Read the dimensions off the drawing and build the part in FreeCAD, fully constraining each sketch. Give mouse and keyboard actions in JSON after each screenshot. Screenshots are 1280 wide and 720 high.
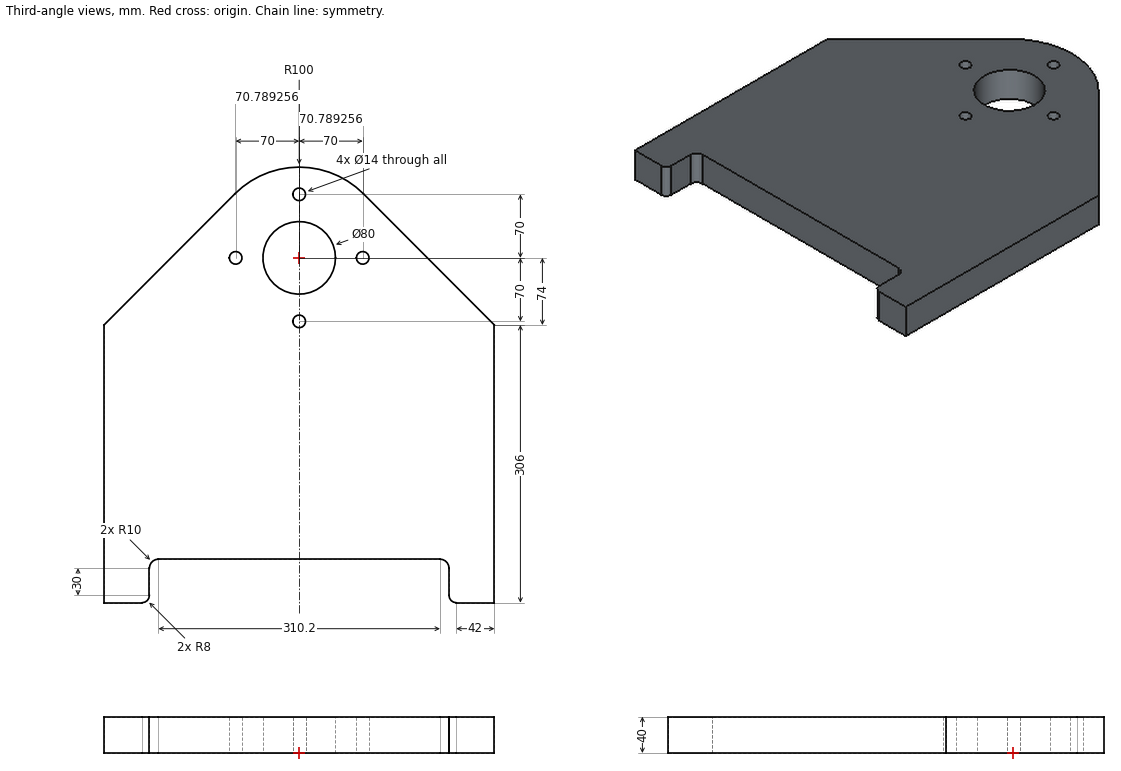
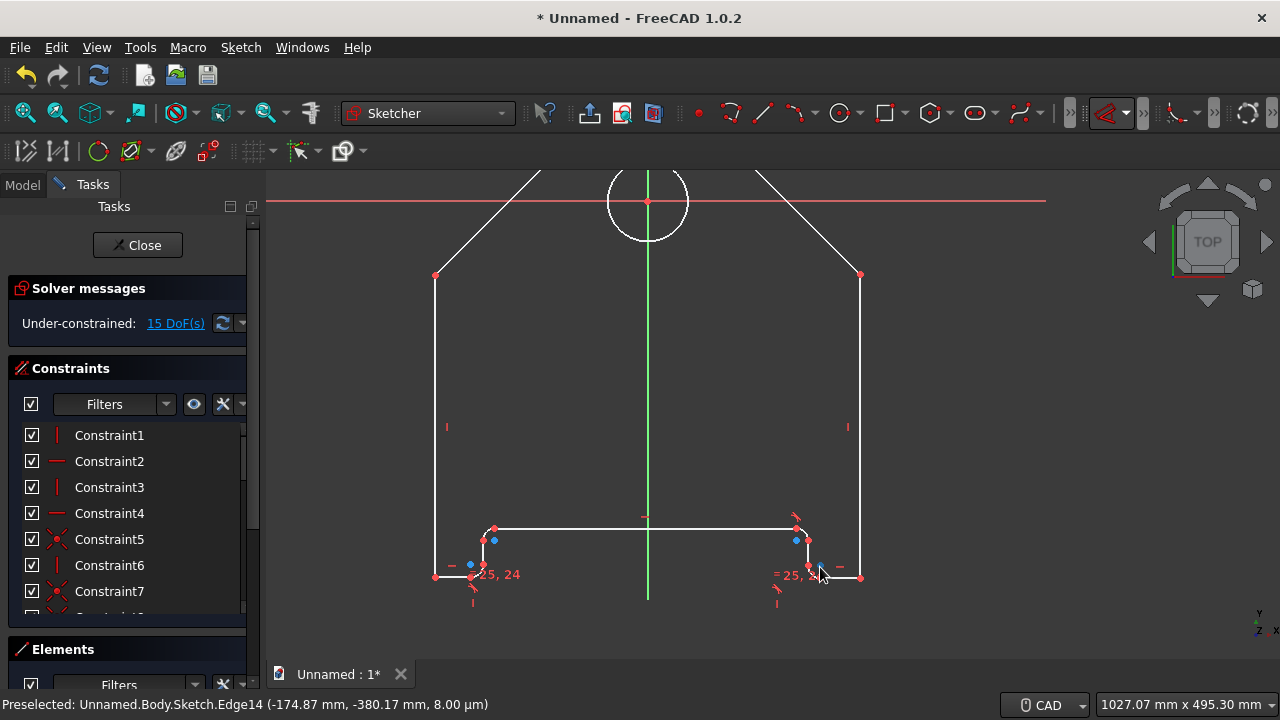
{"action": "left_click", "coordinate": [820, 566]}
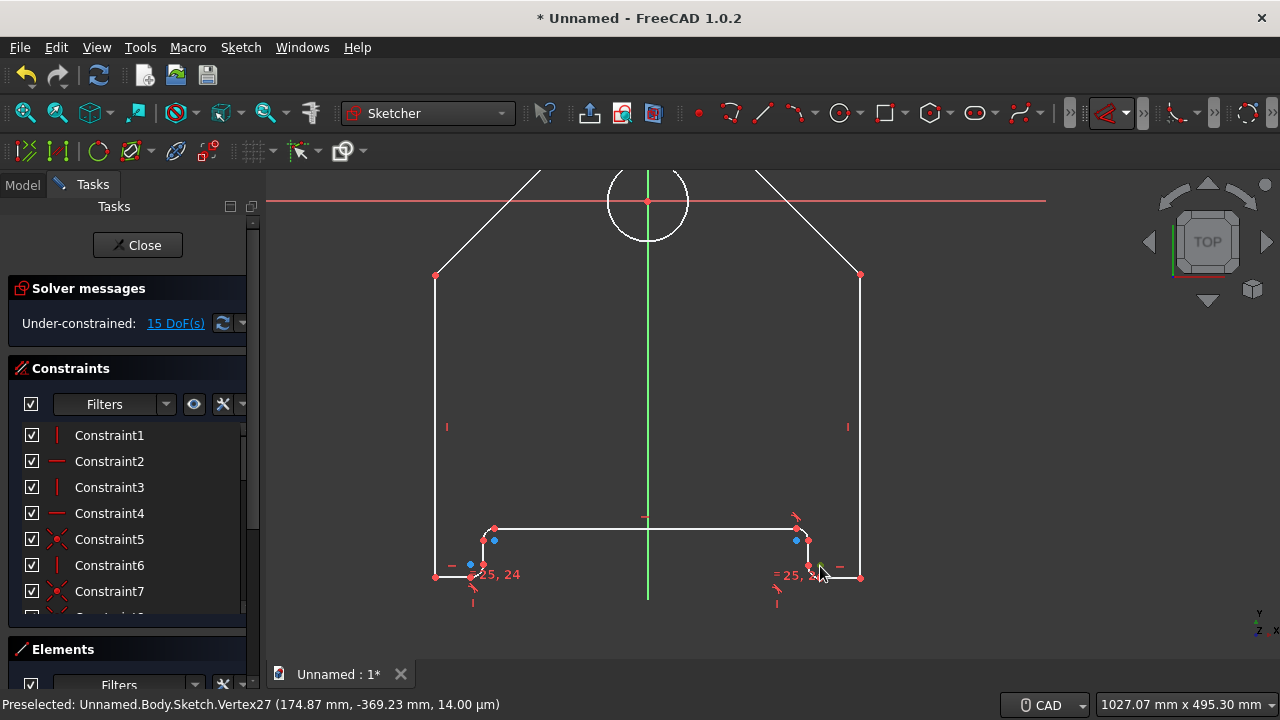
{"action": "left_click", "coordinate": [471, 565]}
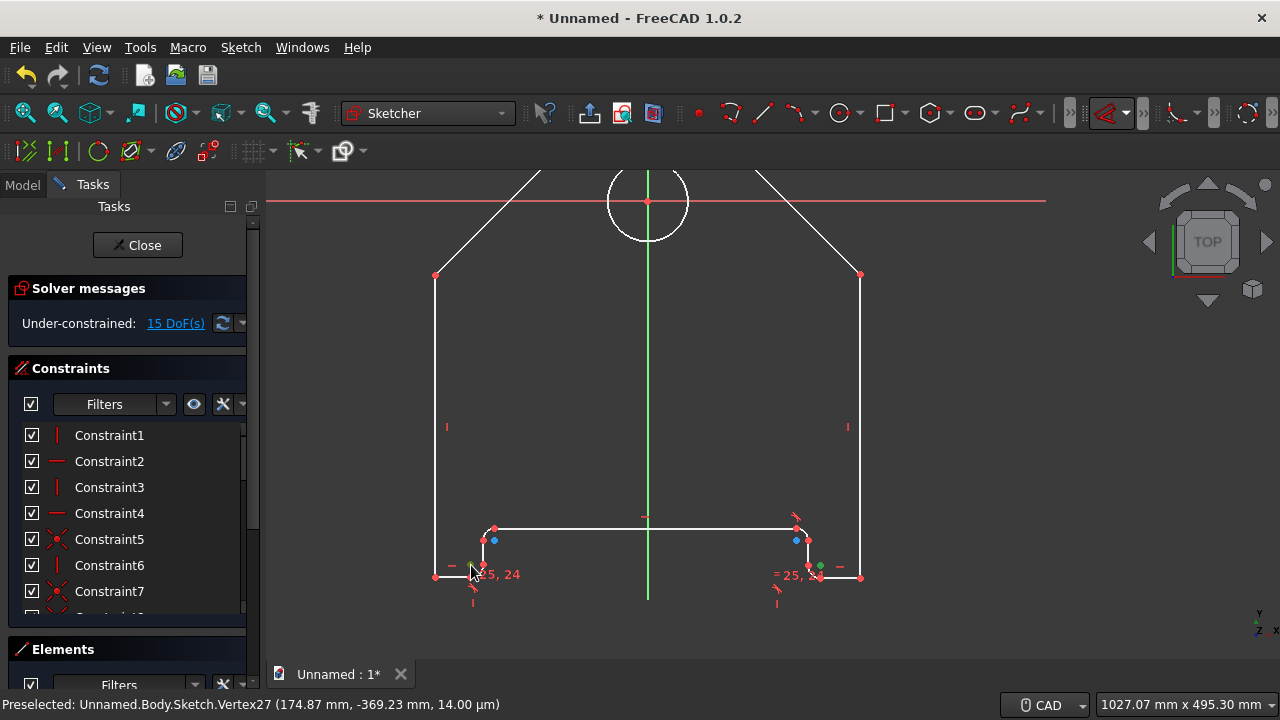
{"action": "left_click", "coordinate": [648, 600]}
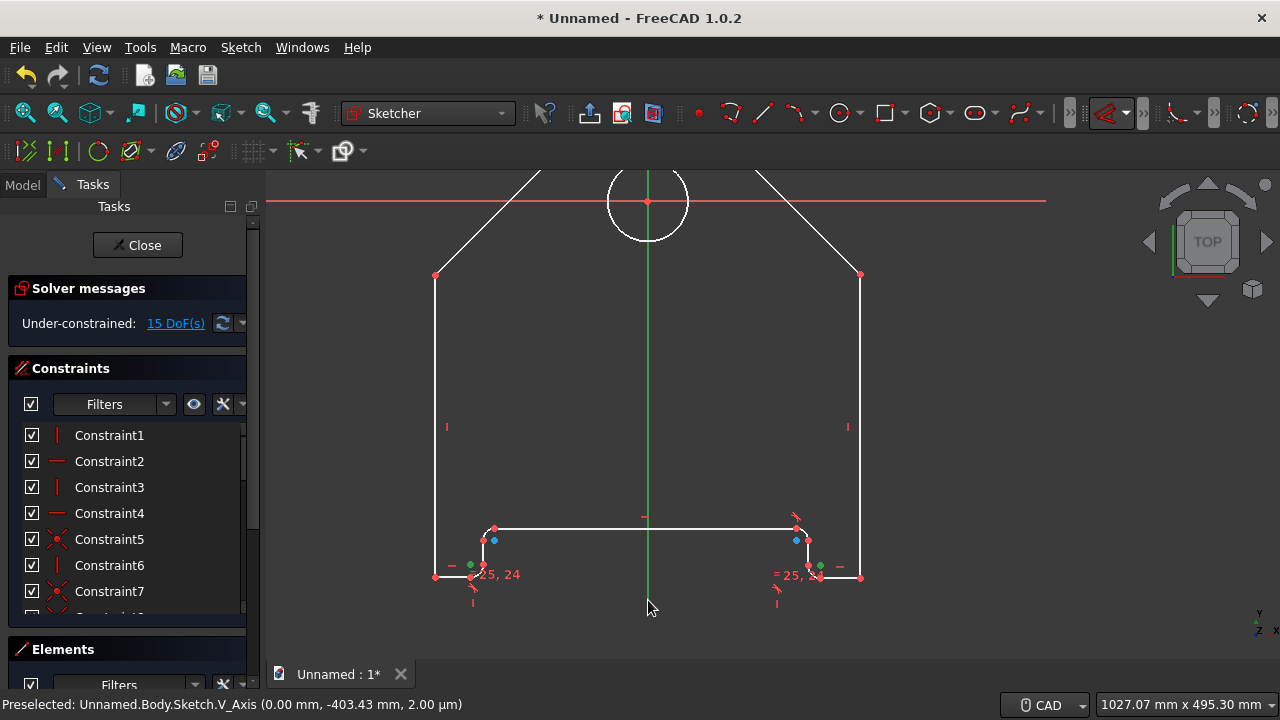
{"action": "key", "text": "s"}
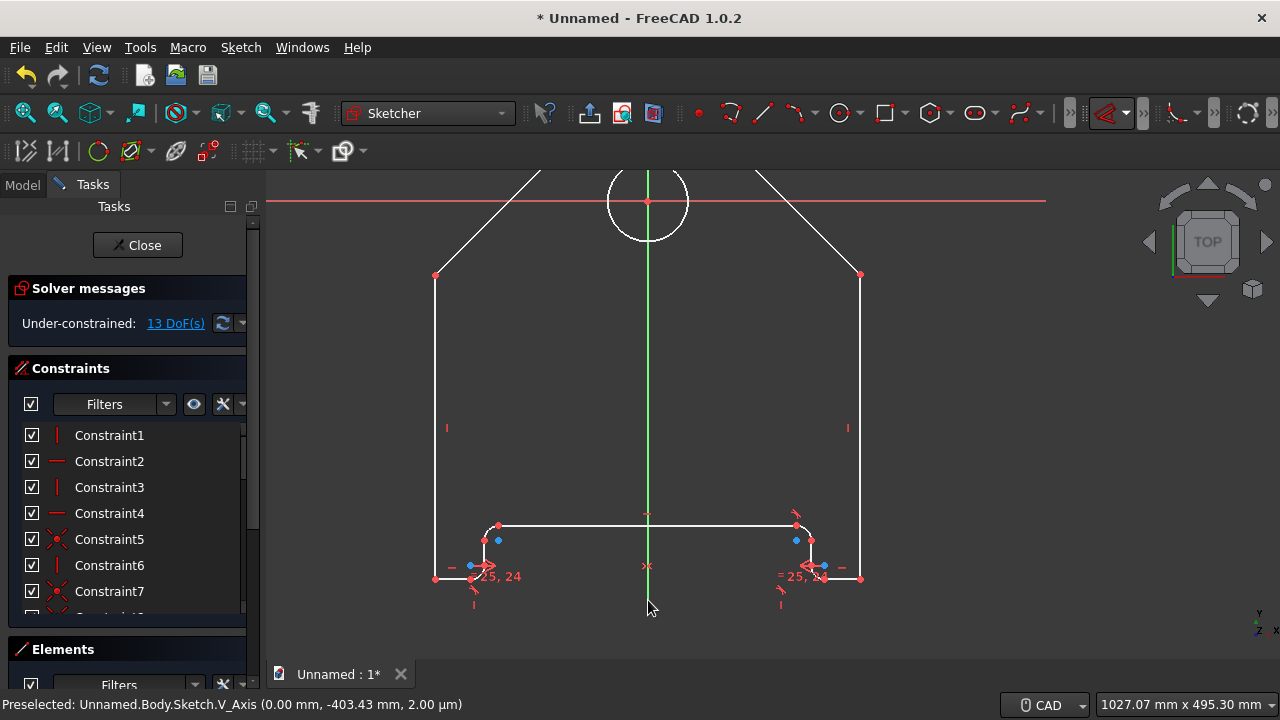
{"action": "left_click", "coordinate": [860, 275]}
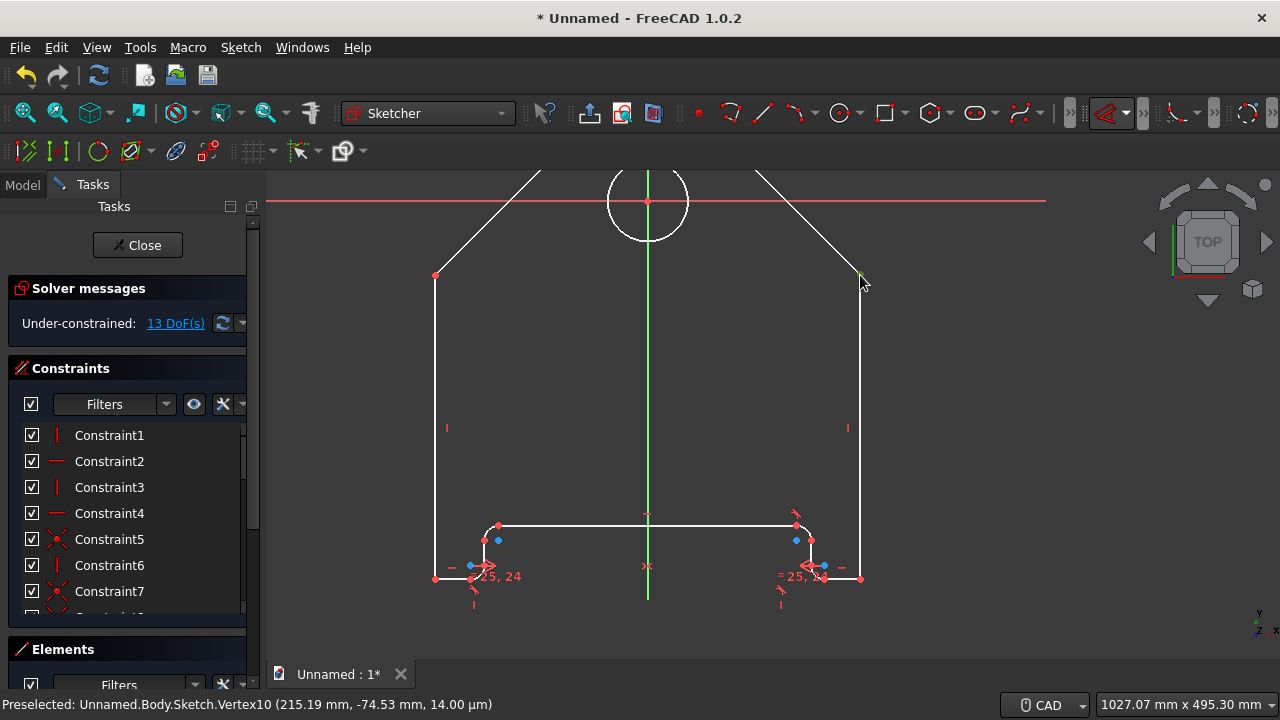
{"action": "left_click", "coordinate": [435, 276]}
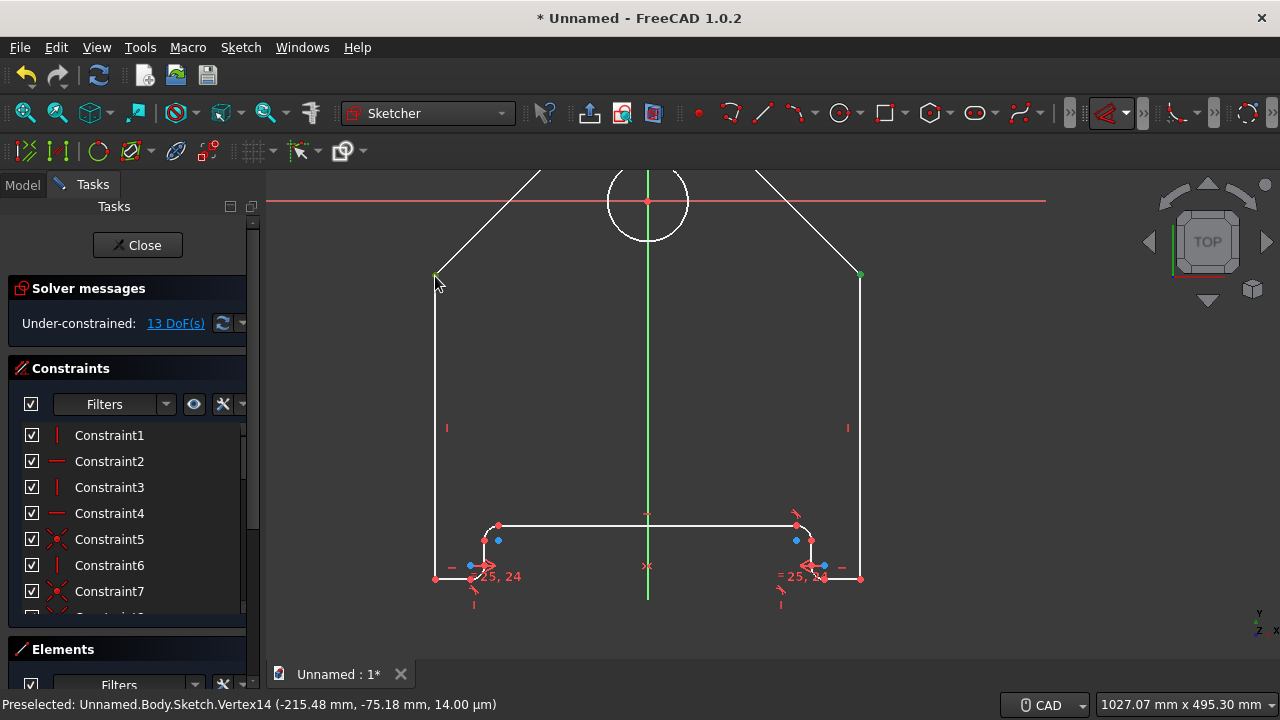
{"action": "left_click", "coordinate": [648, 600]}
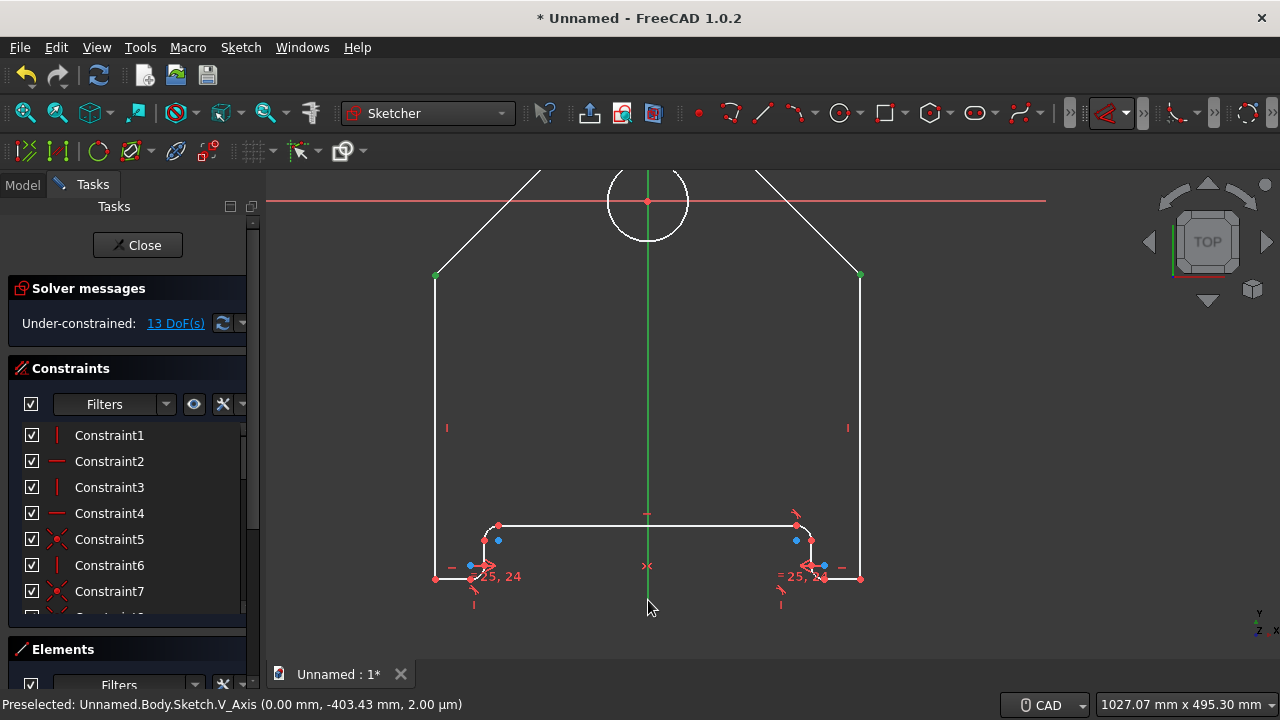
{"action": "key", "text": "s"}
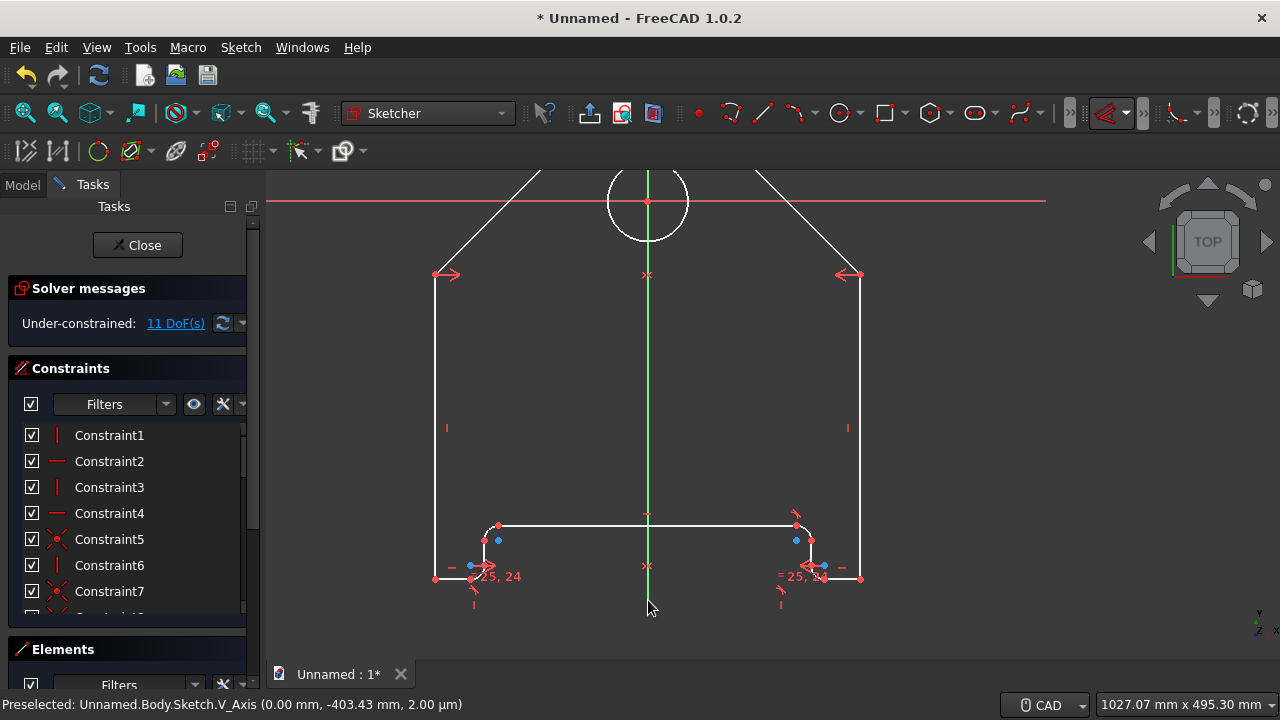
{"action": "key", "text": "d"}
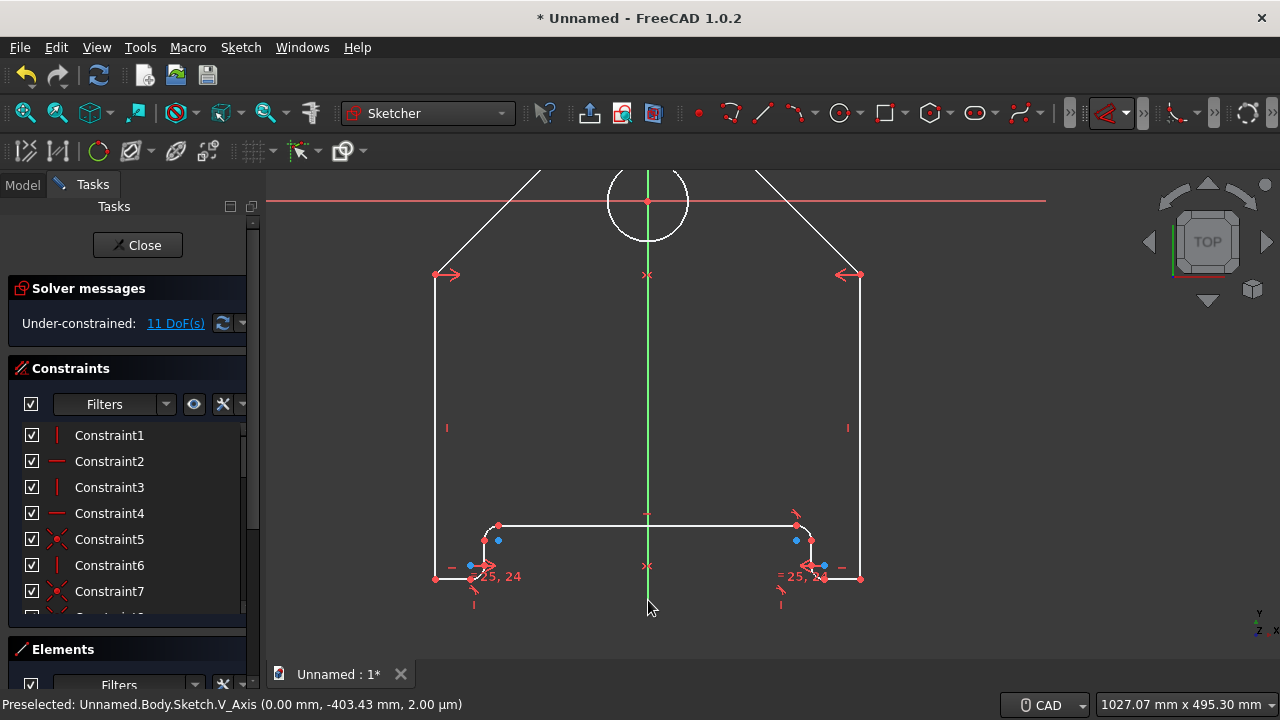
{"action": "scroll", "coordinate": [489, 530], "scroll_direction": "up", "scroll_amount": 7}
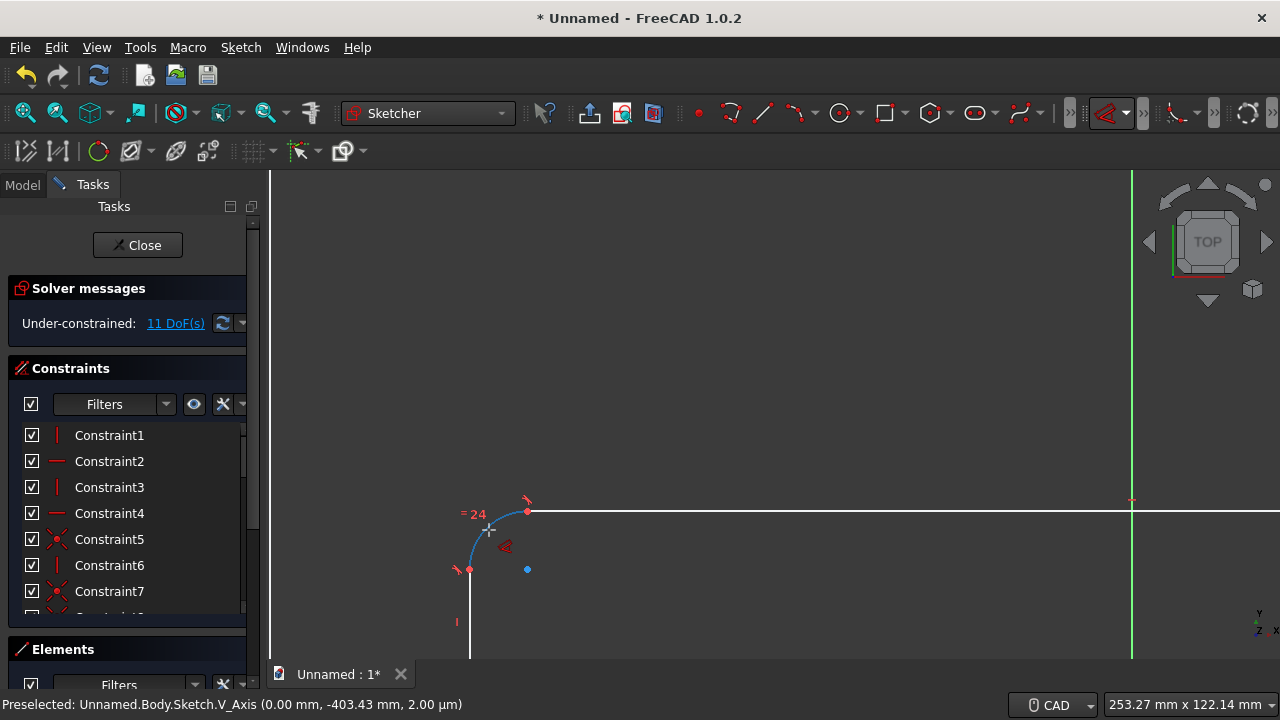
{"action": "left_click", "coordinate": [487, 528]}
{"action": "left_click", "coordinate": [465, 505]}